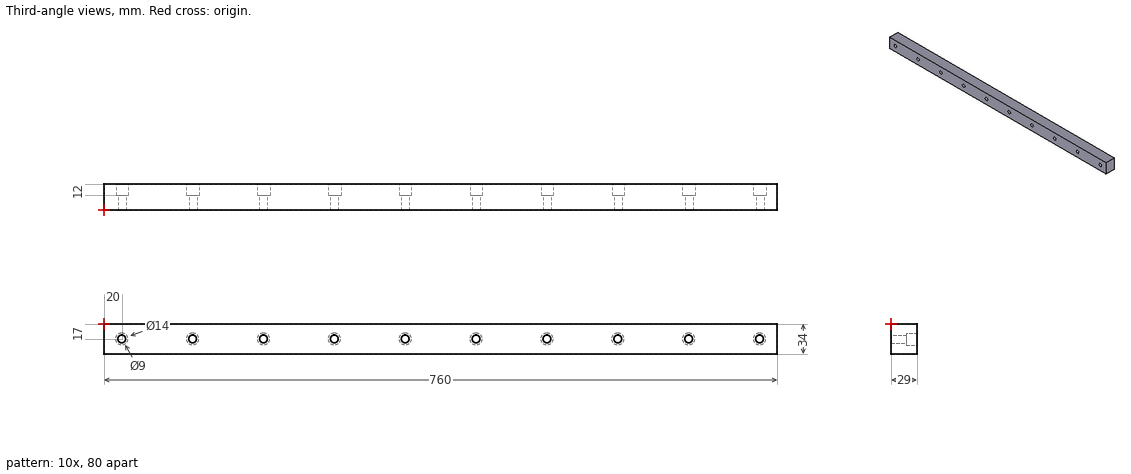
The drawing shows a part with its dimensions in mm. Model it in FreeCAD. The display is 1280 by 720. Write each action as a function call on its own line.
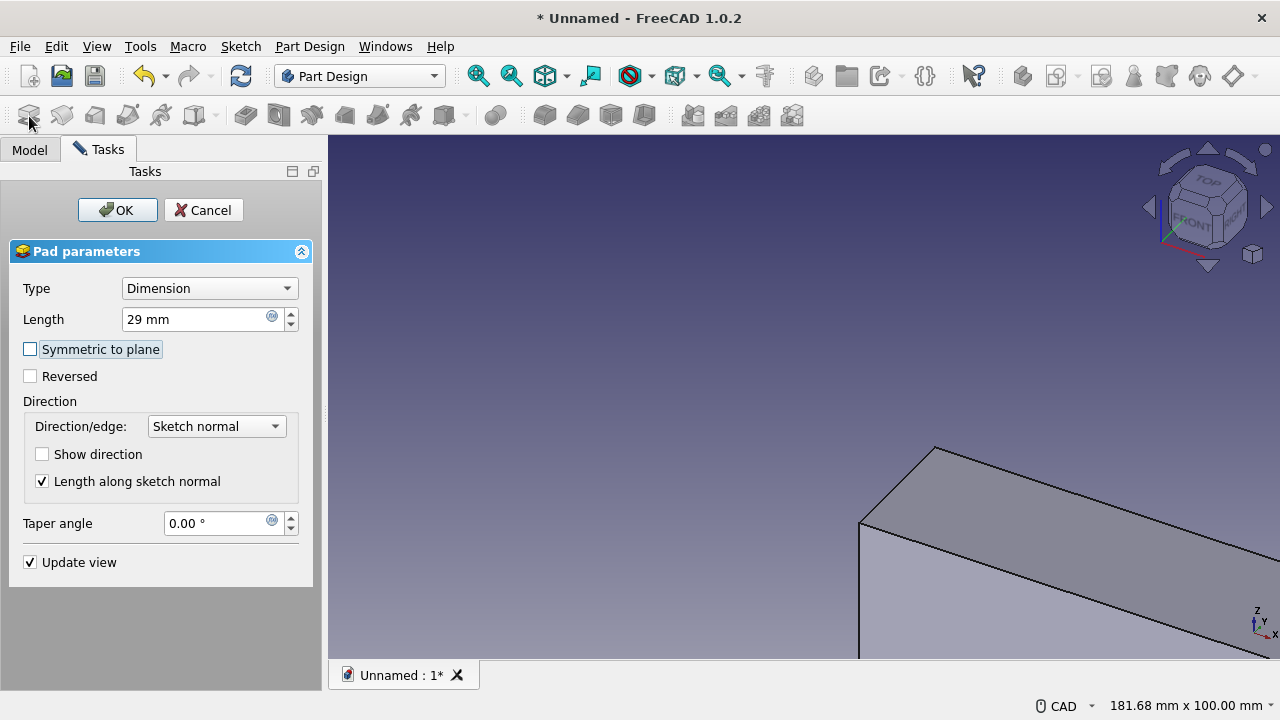
click(31, 376)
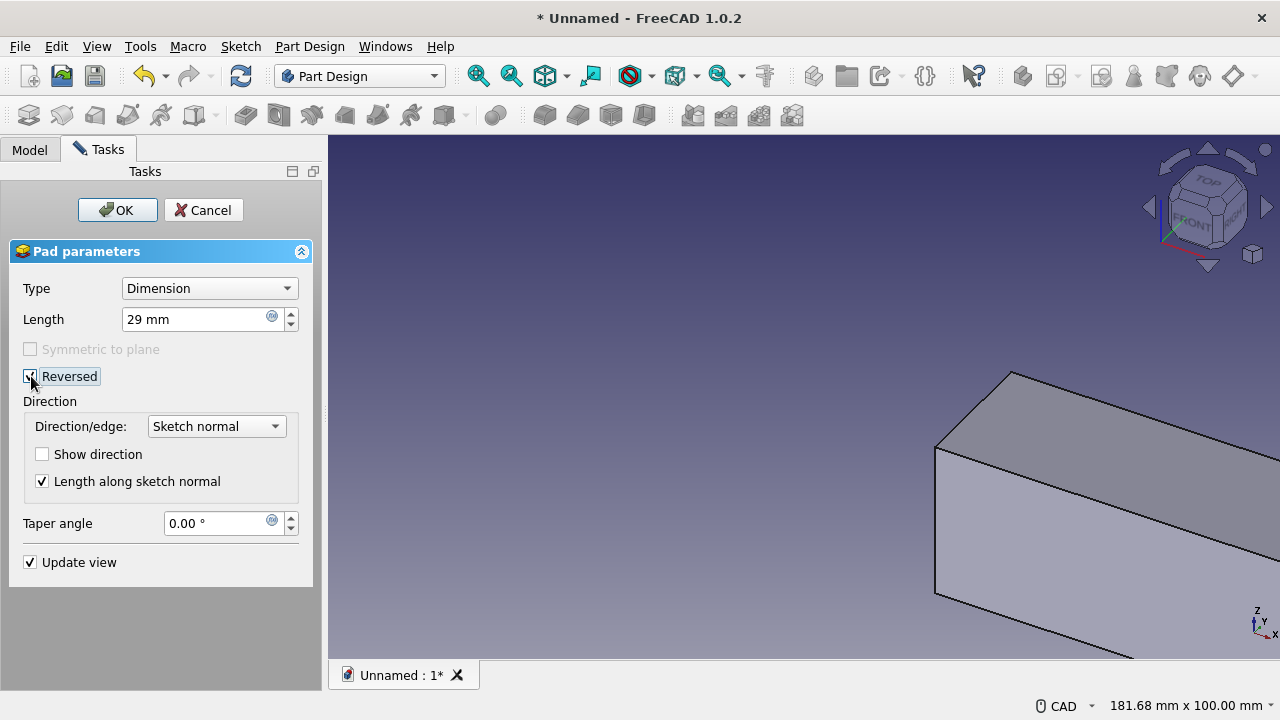
click(118, 210)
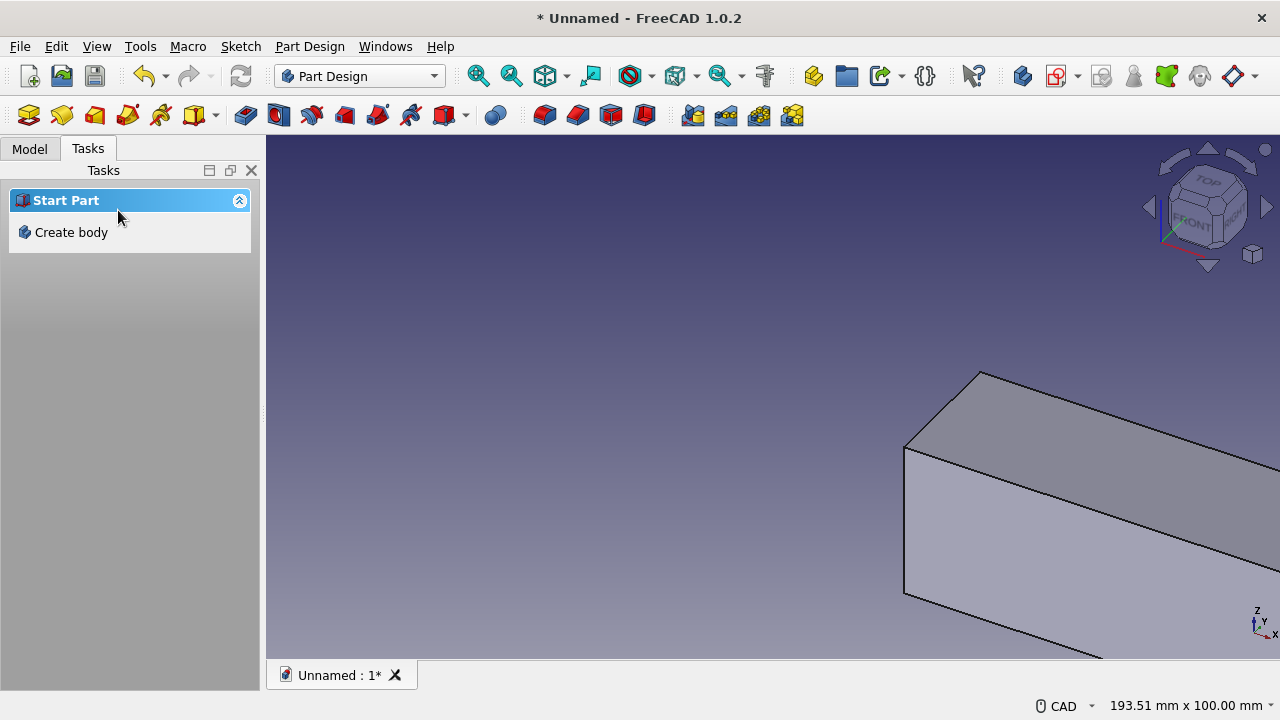
key(v)
key(f)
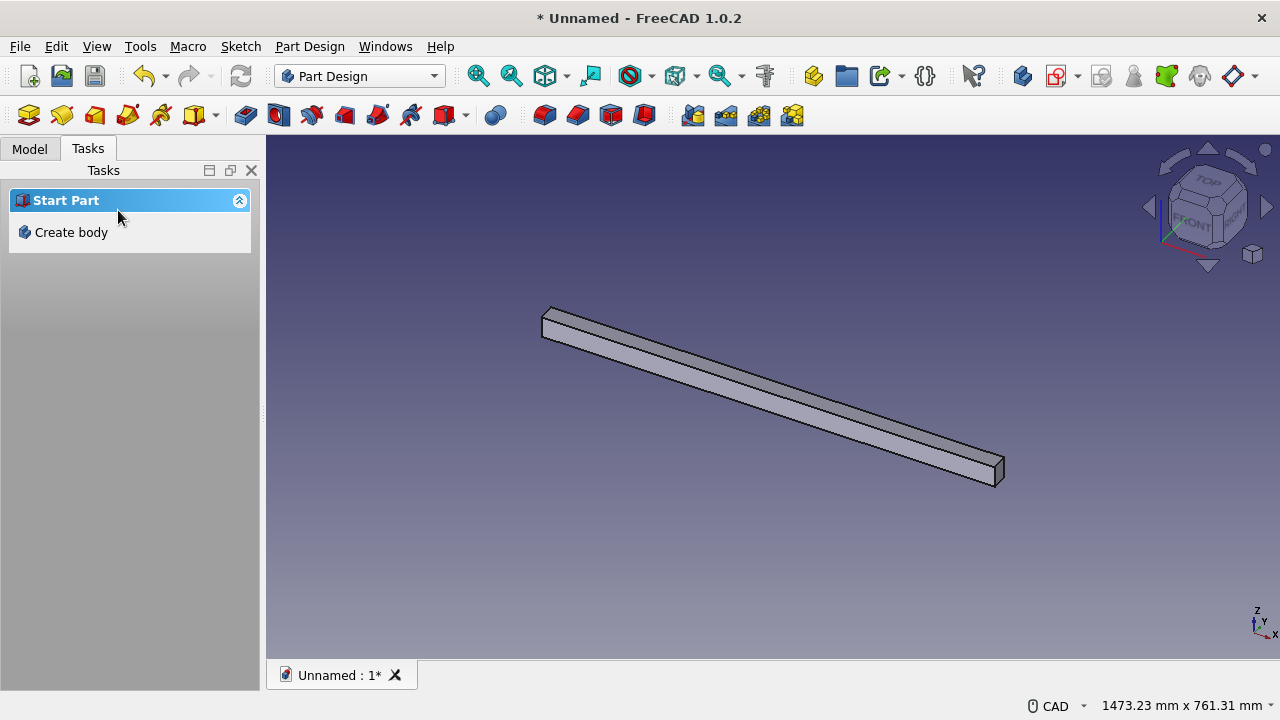
key(4)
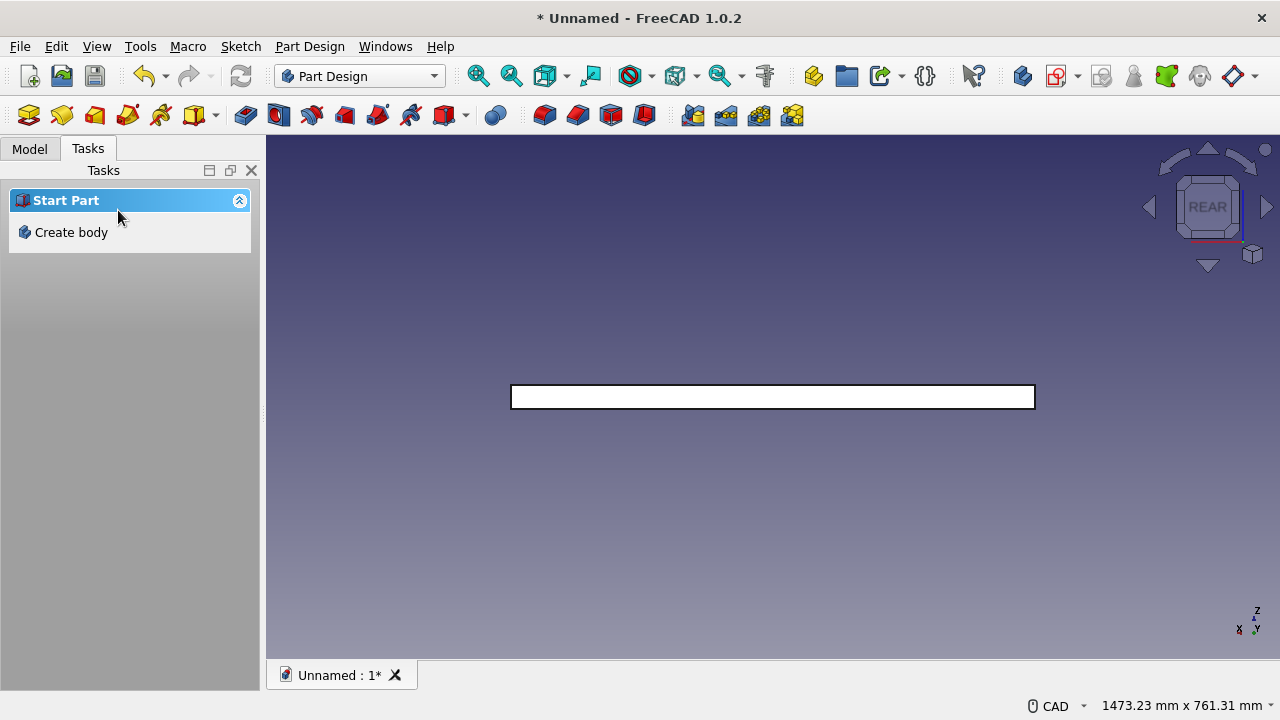
click(549, 396)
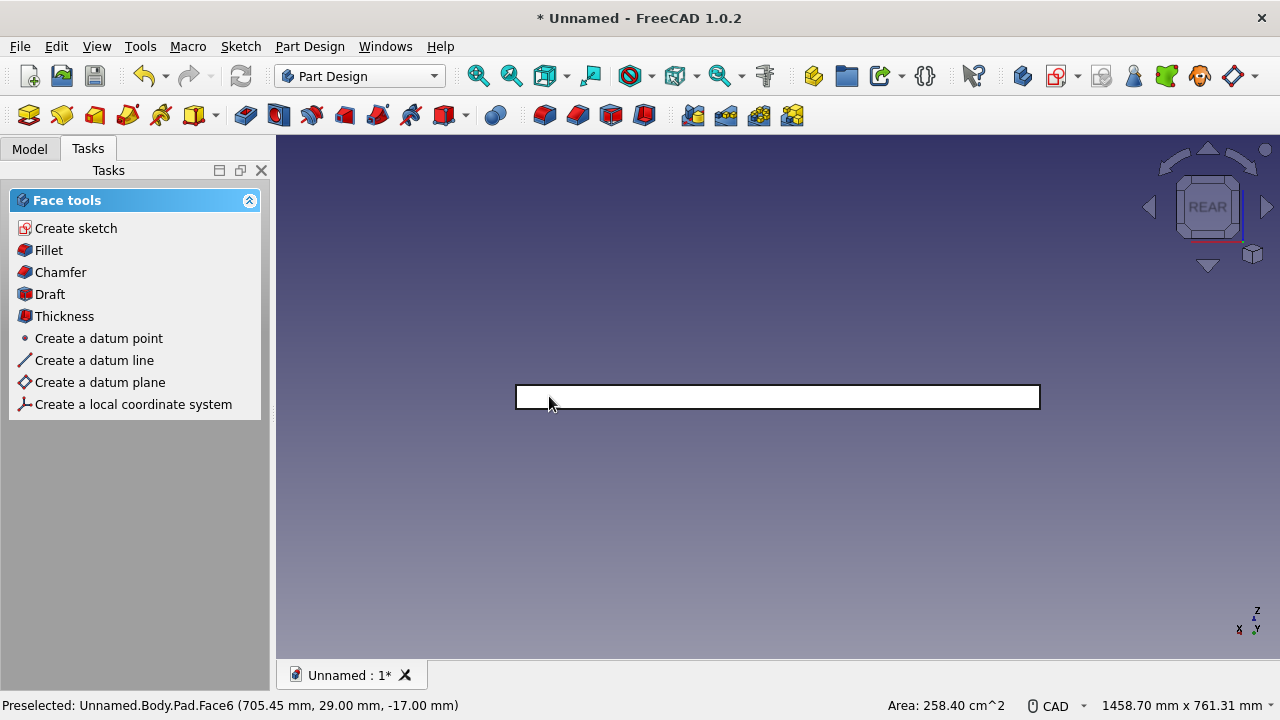
click(1056, 76)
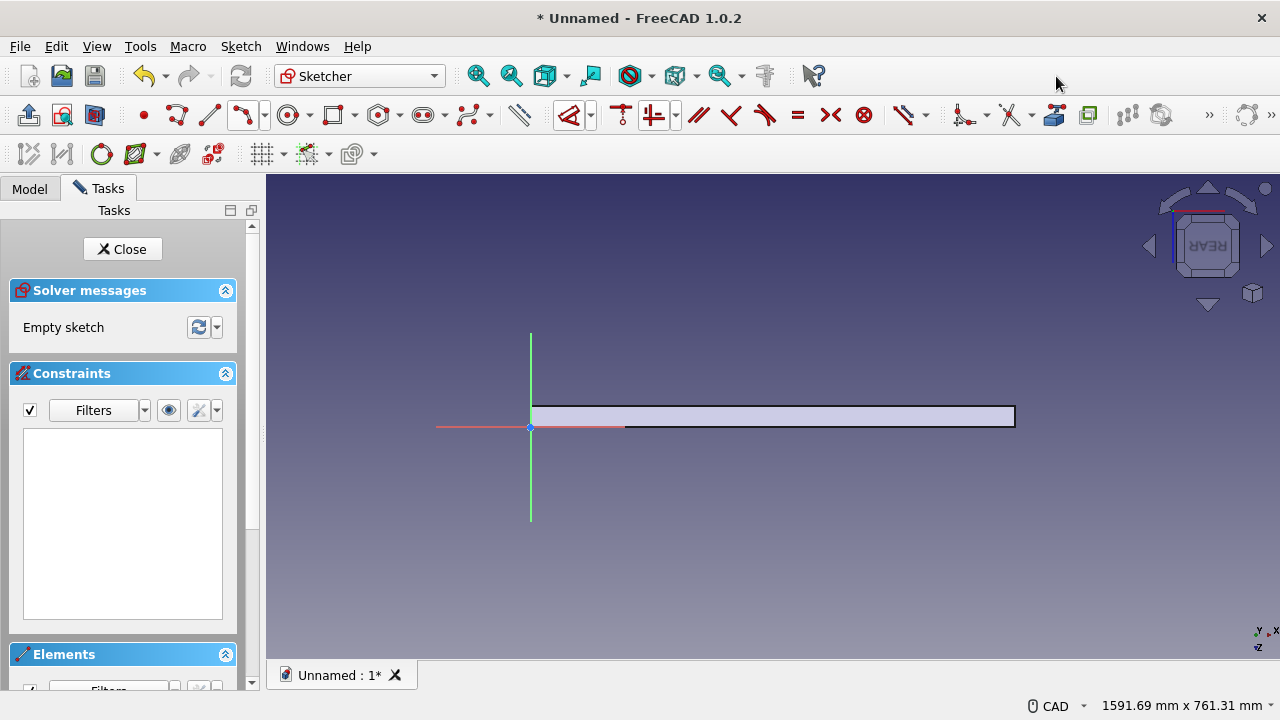
scroll(531, 420, up, 15)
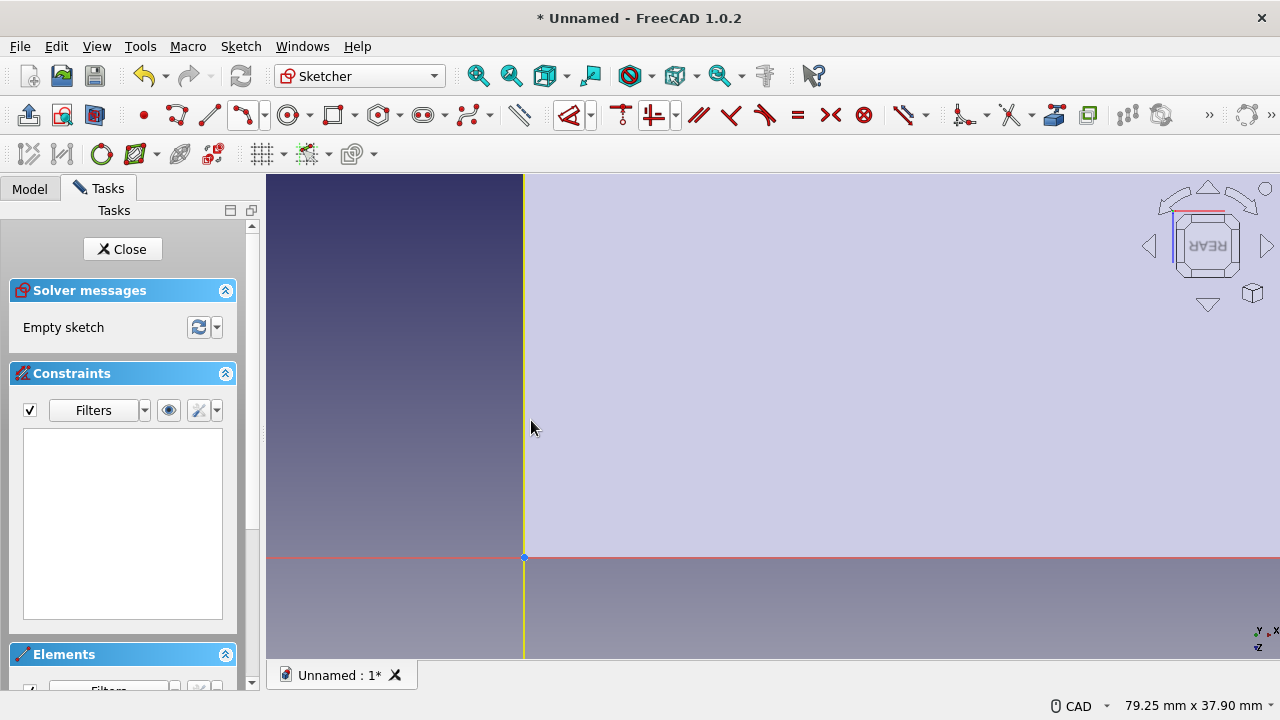
key(g)
key(c)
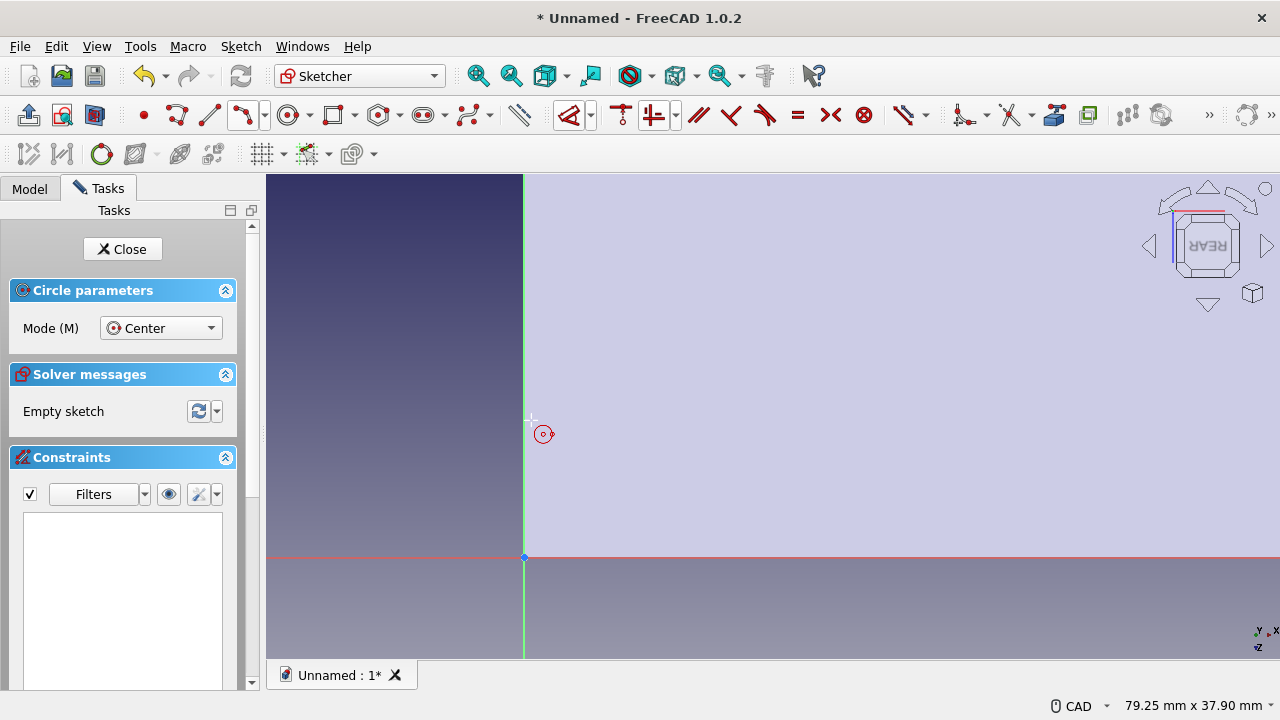
click(780, 340)
move(844, 277)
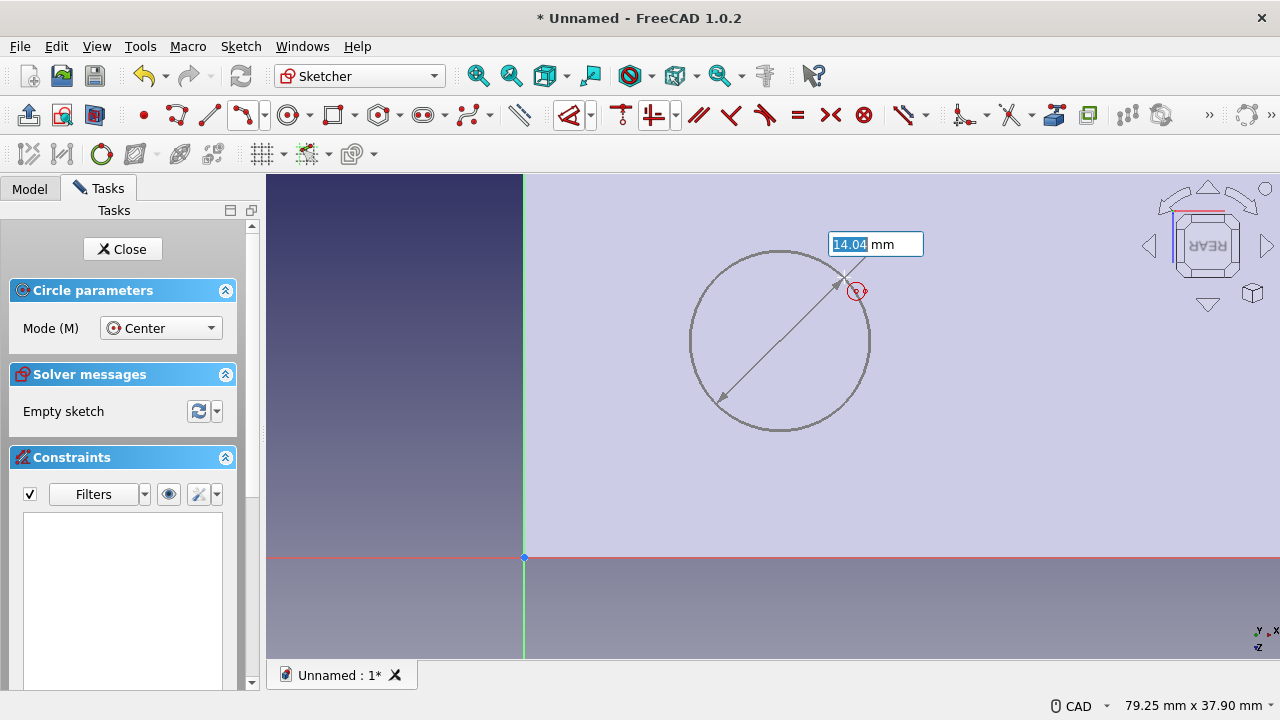
text(14)
key(Return)
key(Escape)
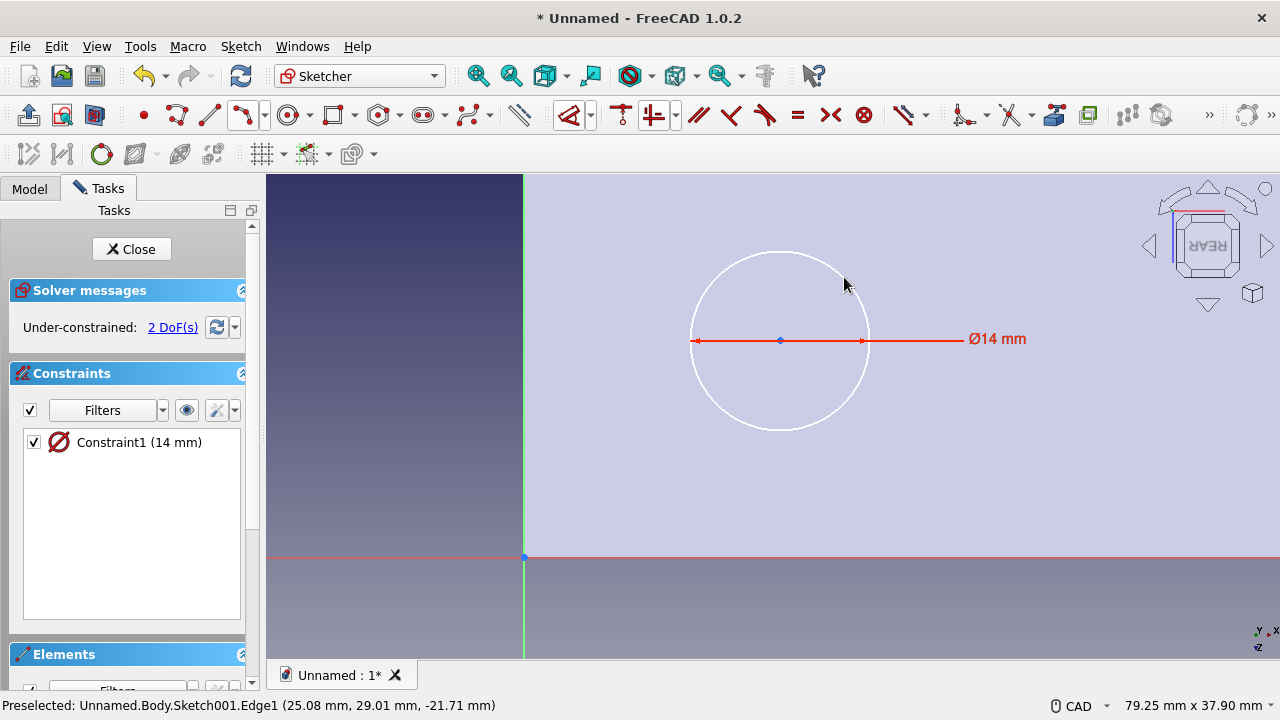
key(d)